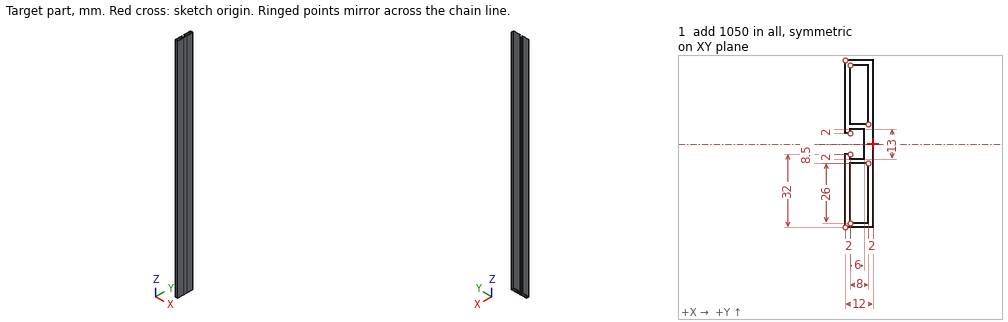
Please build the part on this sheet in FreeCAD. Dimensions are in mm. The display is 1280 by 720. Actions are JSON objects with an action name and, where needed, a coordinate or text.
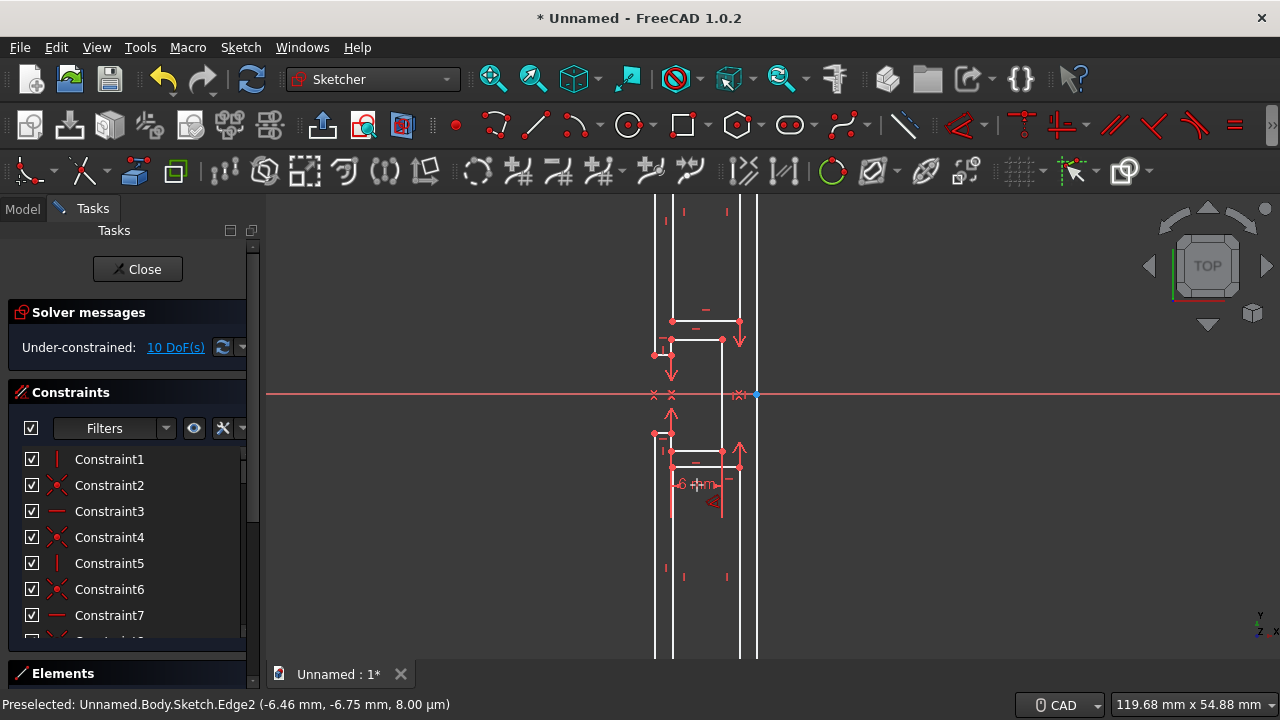
{"action": "scroll", "coordinate": [671, 442], "scroll_direction": "up", "scroll_amount": 5}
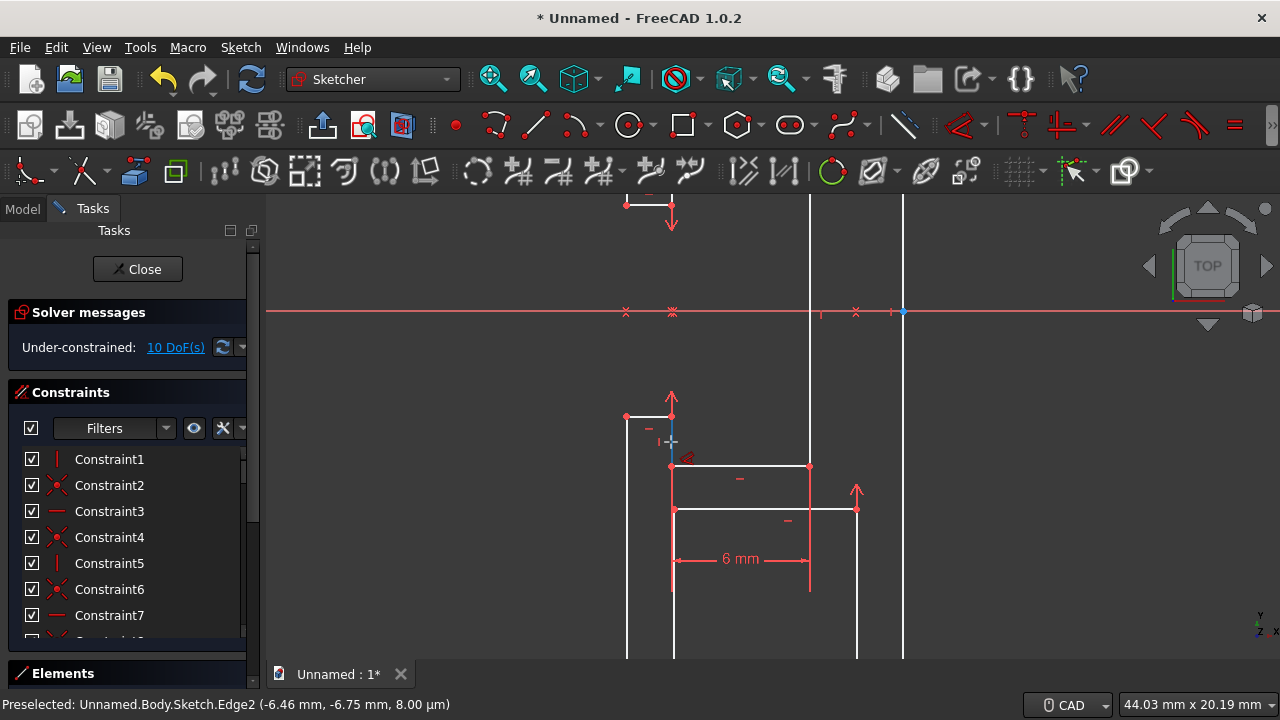
{"action": "left_click", "coordinate": [672, 442]}
{"action": "left_click", "coordinate": [706, 442]}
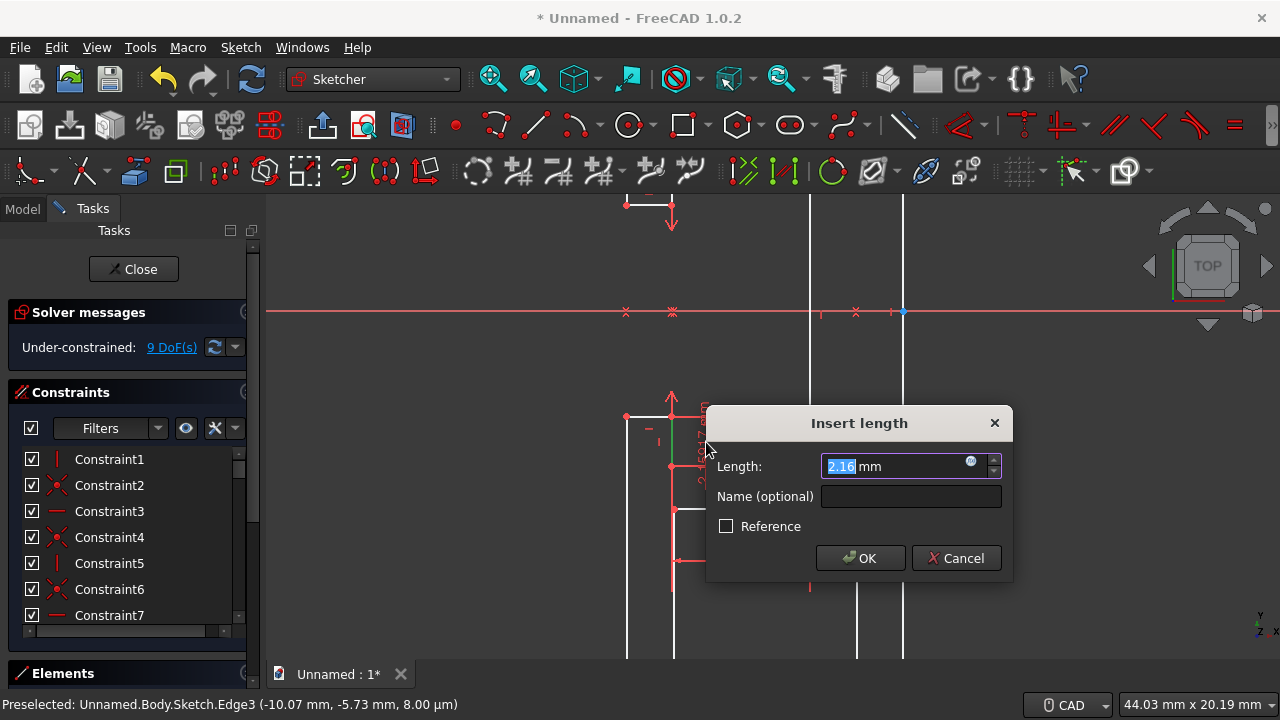
{"action": "type", "text": "2"}
{"action": "key", "text": "Return"}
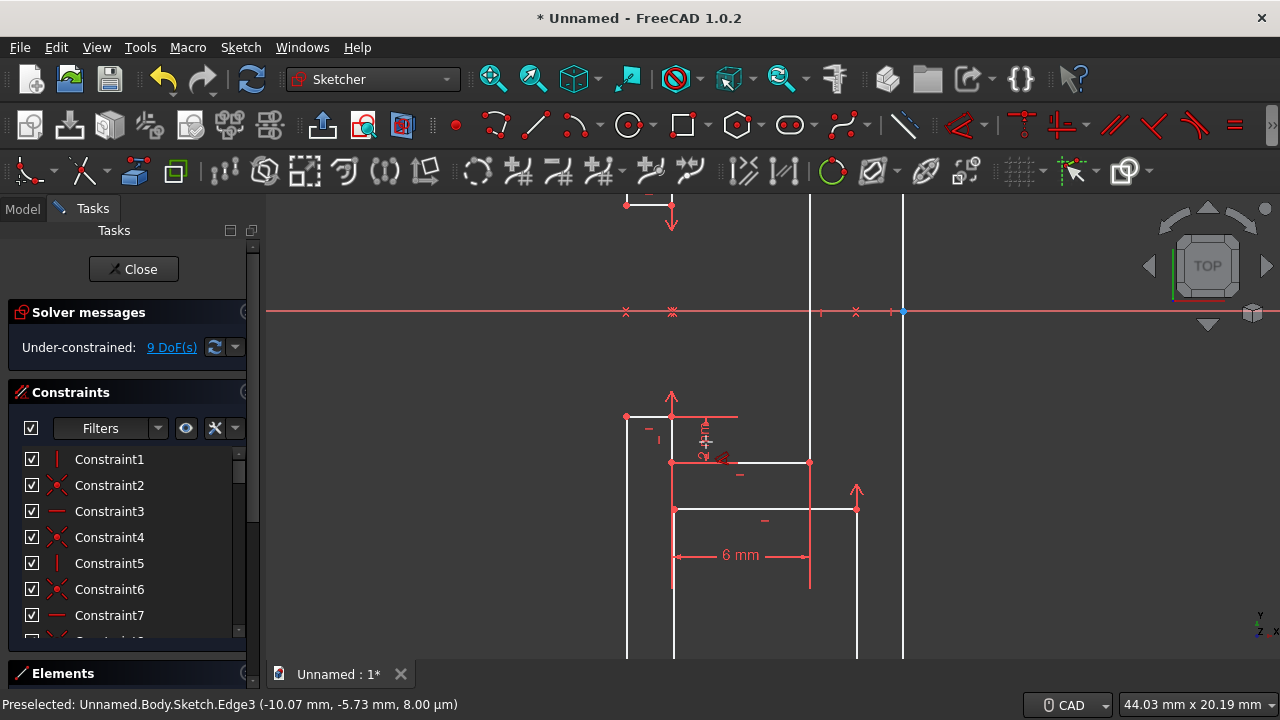
{"action": "left_click", "coordinate": [658, 417]}
{"action": "left_click", "coordinate": [649, 383]}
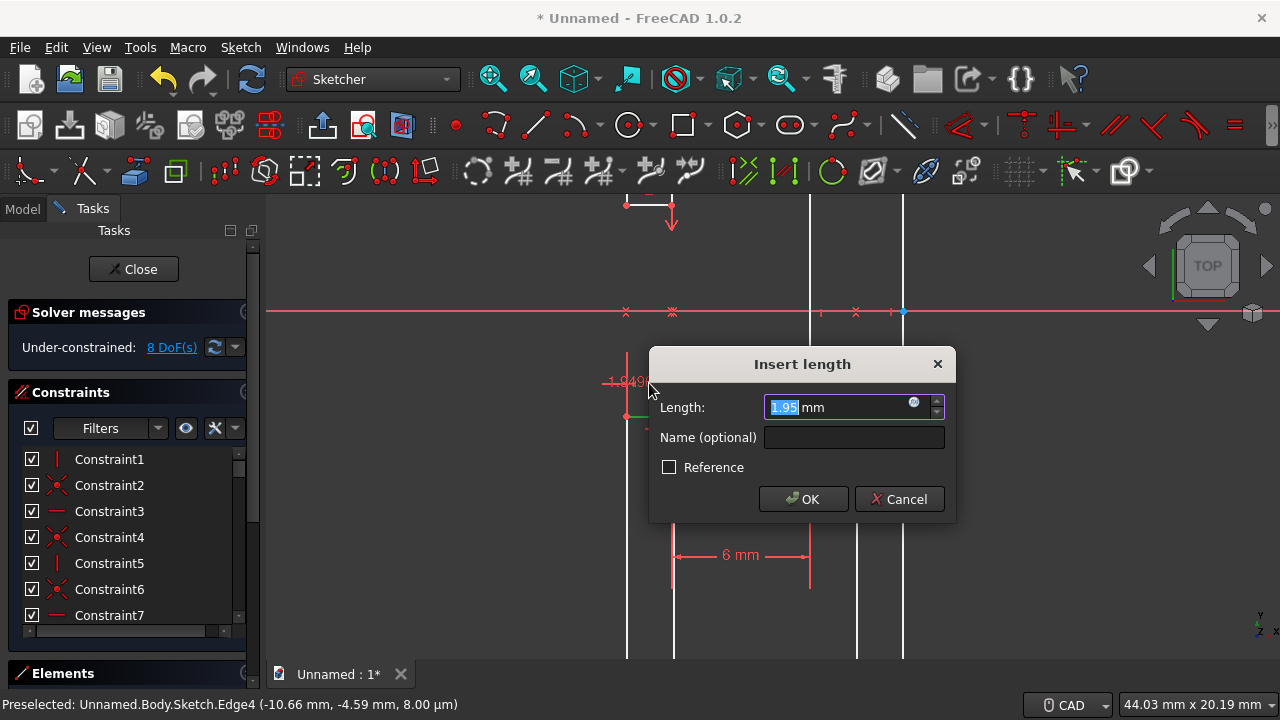
{"action": "type", "text": "2"}
{"action": "key", "text": "Return"}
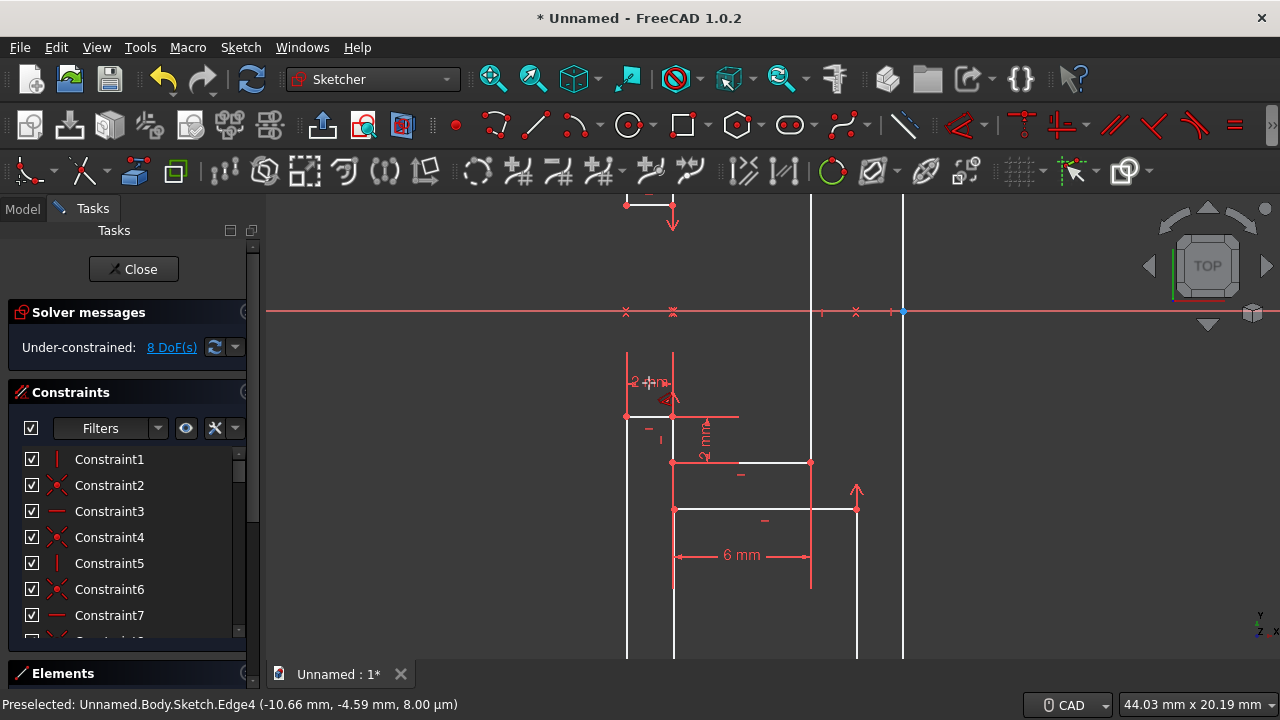
{"action": "scroll", "coordinate": [692, 449], "scroll_direction": "down", "scroll_amount": 9}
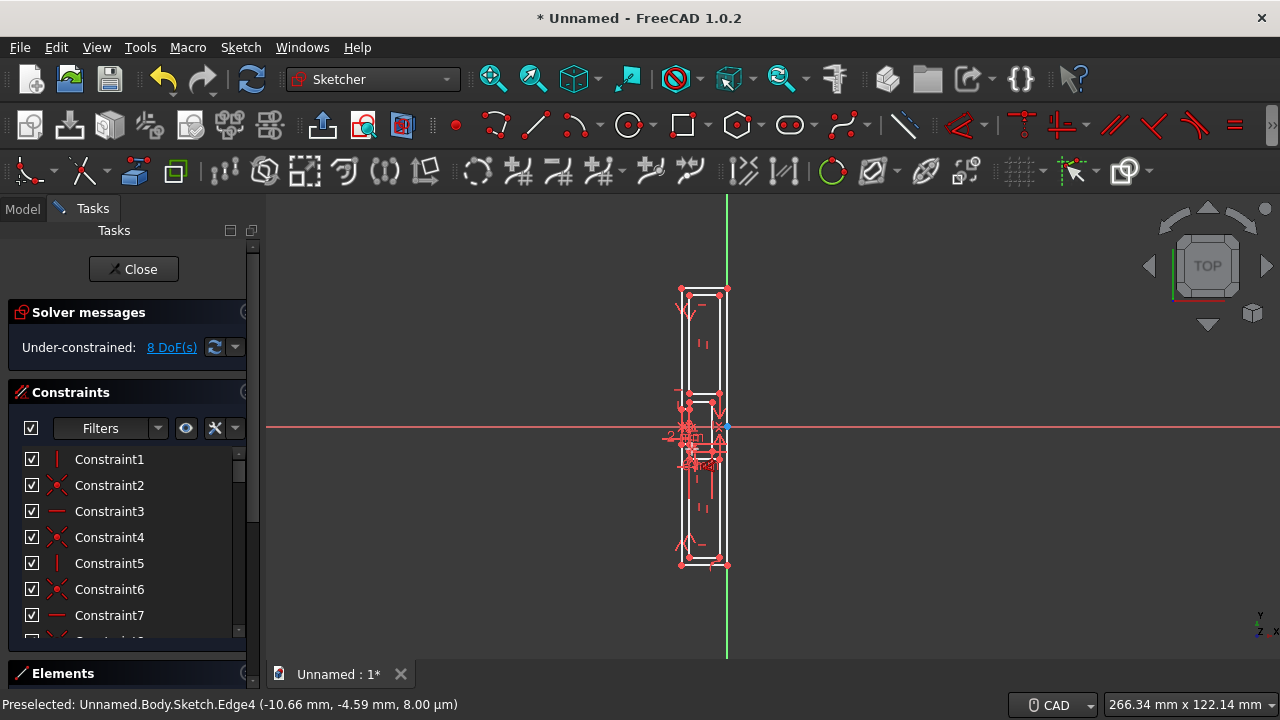
{"action": "scroll", "coordinate": [689, 407], "scroll_direction": "up", "scroll_amount": 10}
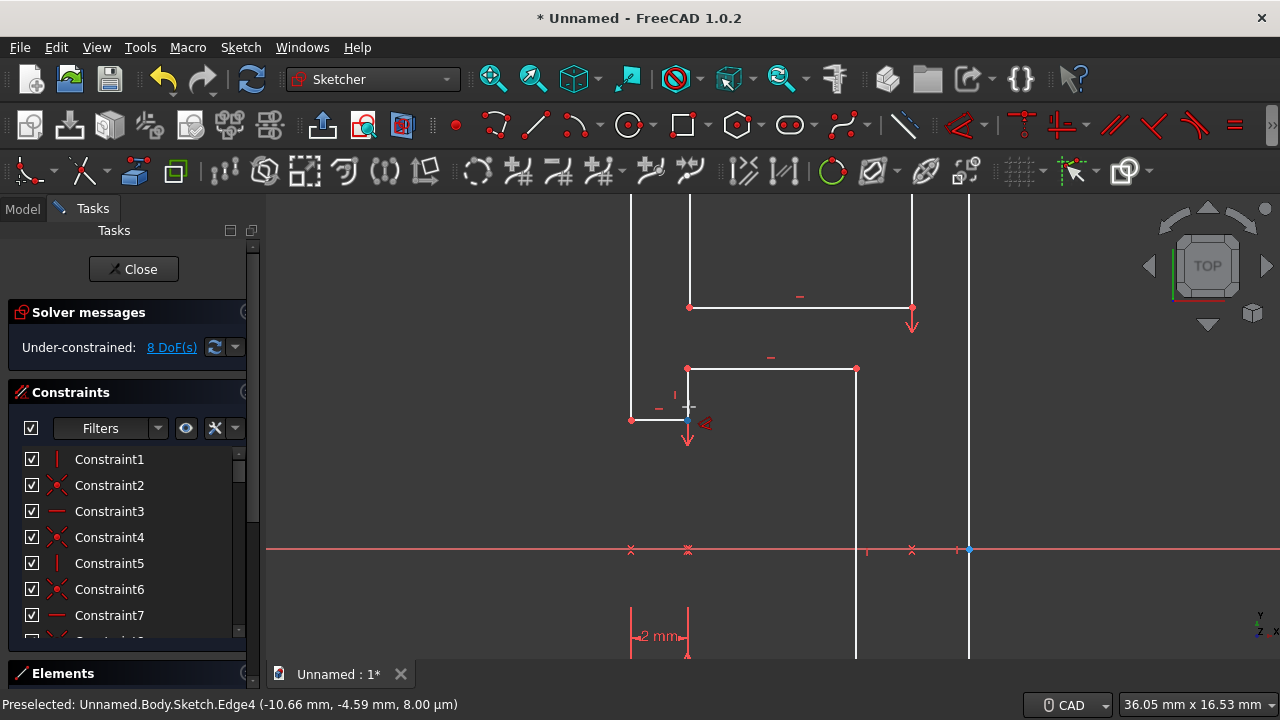
{"action": "left_click", "coordinate": [688, 405]}
{"action": "left_click", "coordinate": [654, 395]}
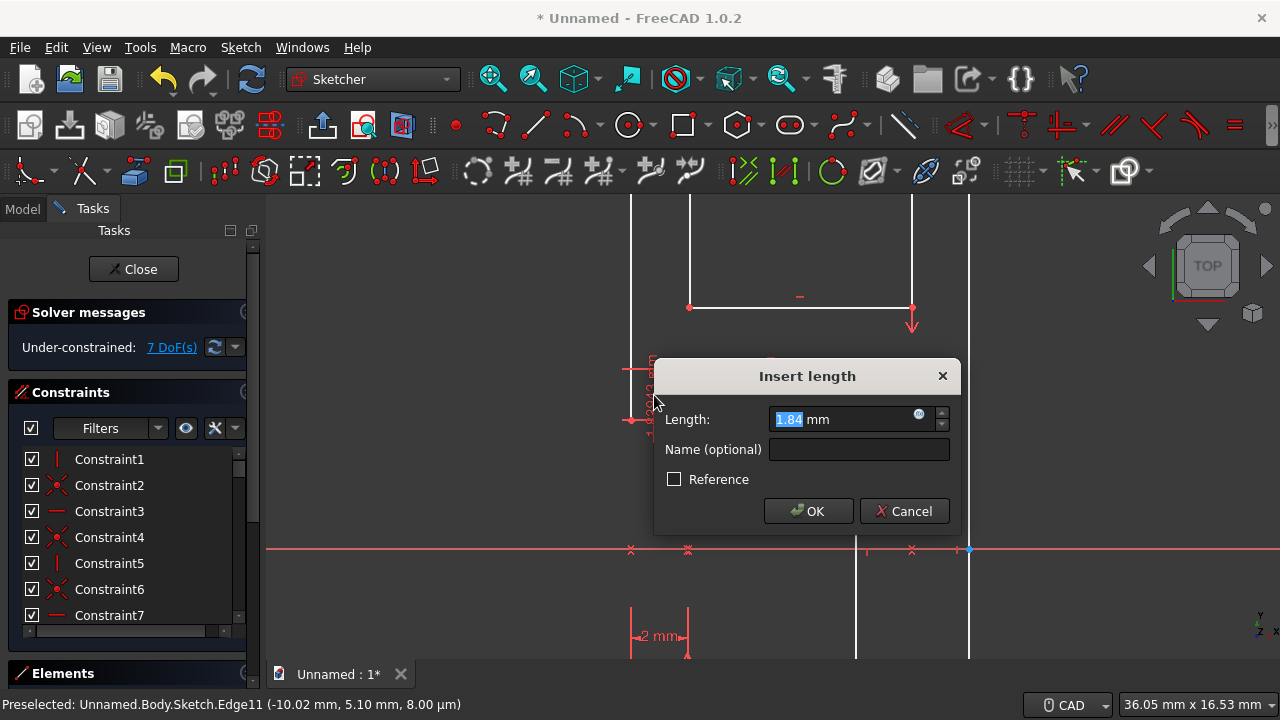
{"action": "type", "text": "2"}
{"action": "key", "text": "Return"}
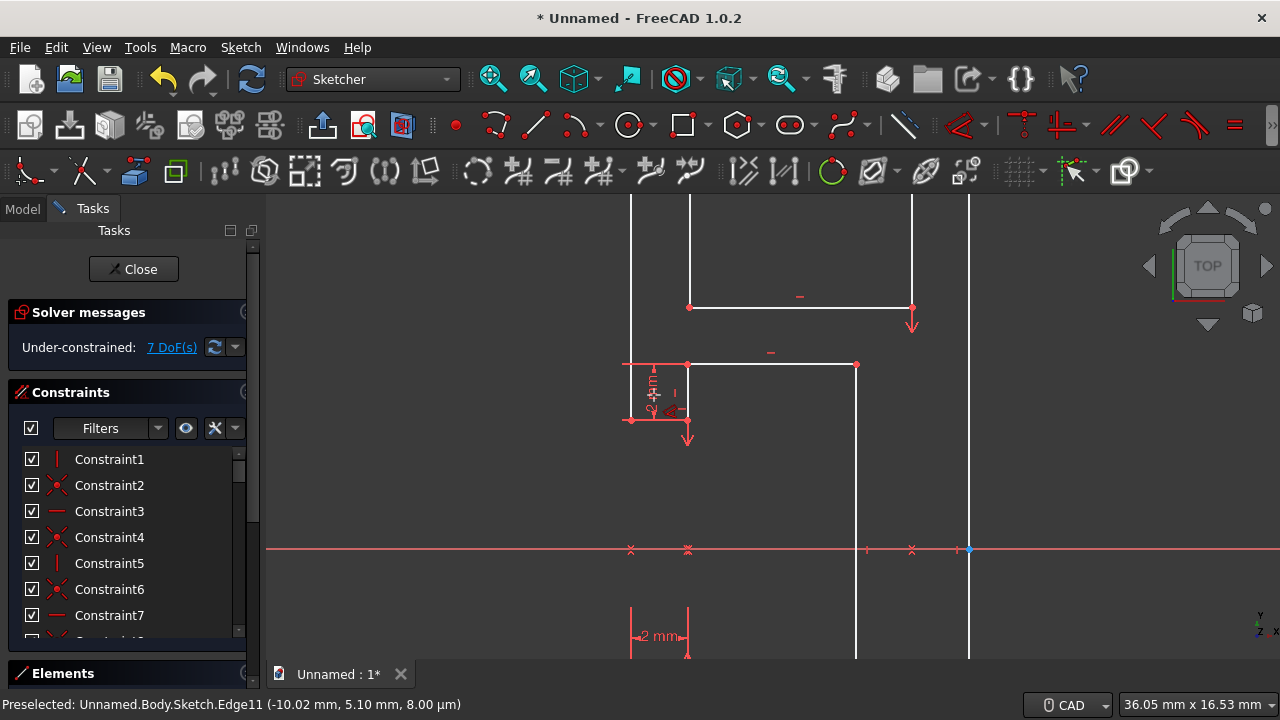
{"action": "scroll", "coordinate": [689, 407], "scroll_direction": "down", "scroll_amount": 10}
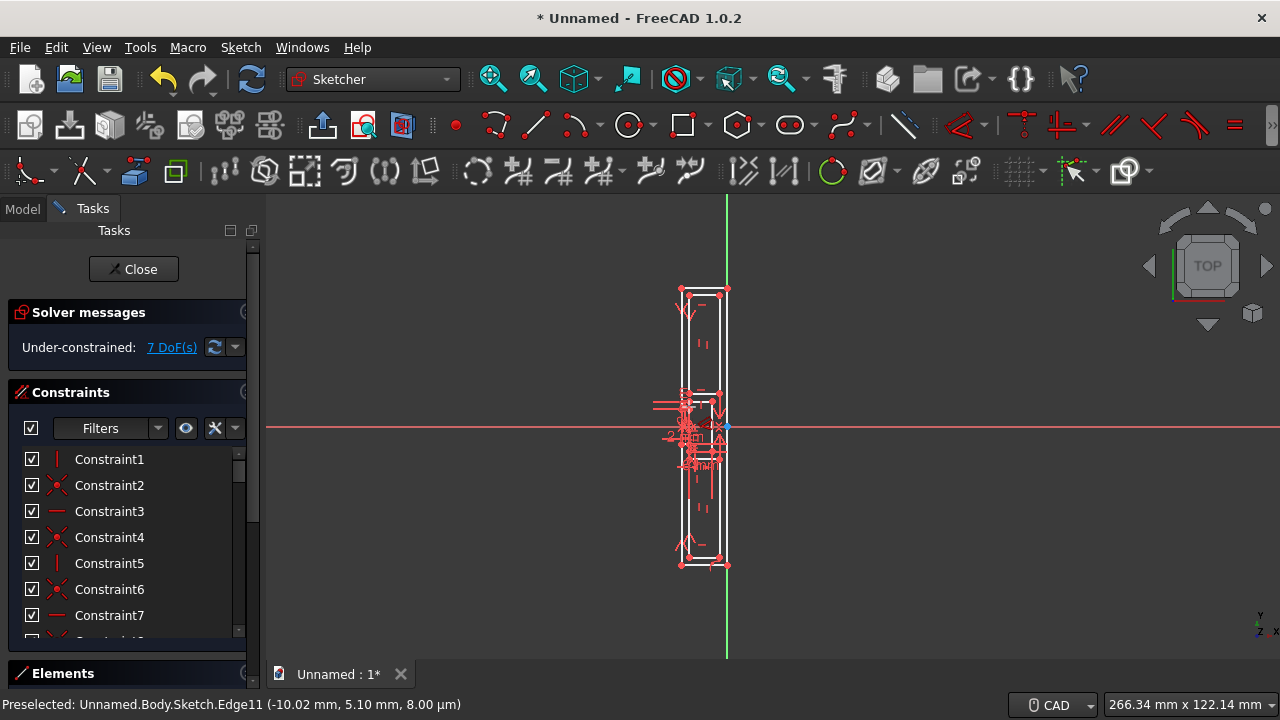
{"action": "scroll", "coordinate": [698, 558], "scroll_direction": "up", "scroll_amount": 4}